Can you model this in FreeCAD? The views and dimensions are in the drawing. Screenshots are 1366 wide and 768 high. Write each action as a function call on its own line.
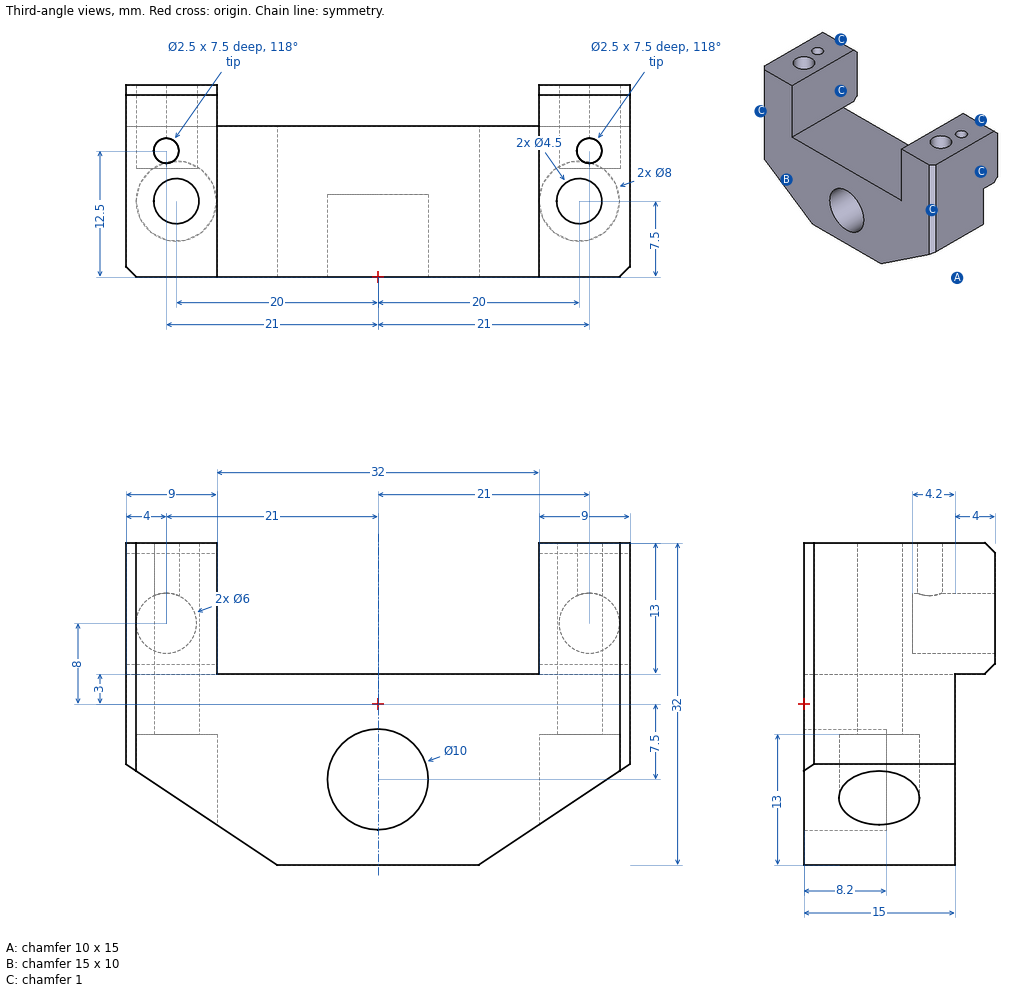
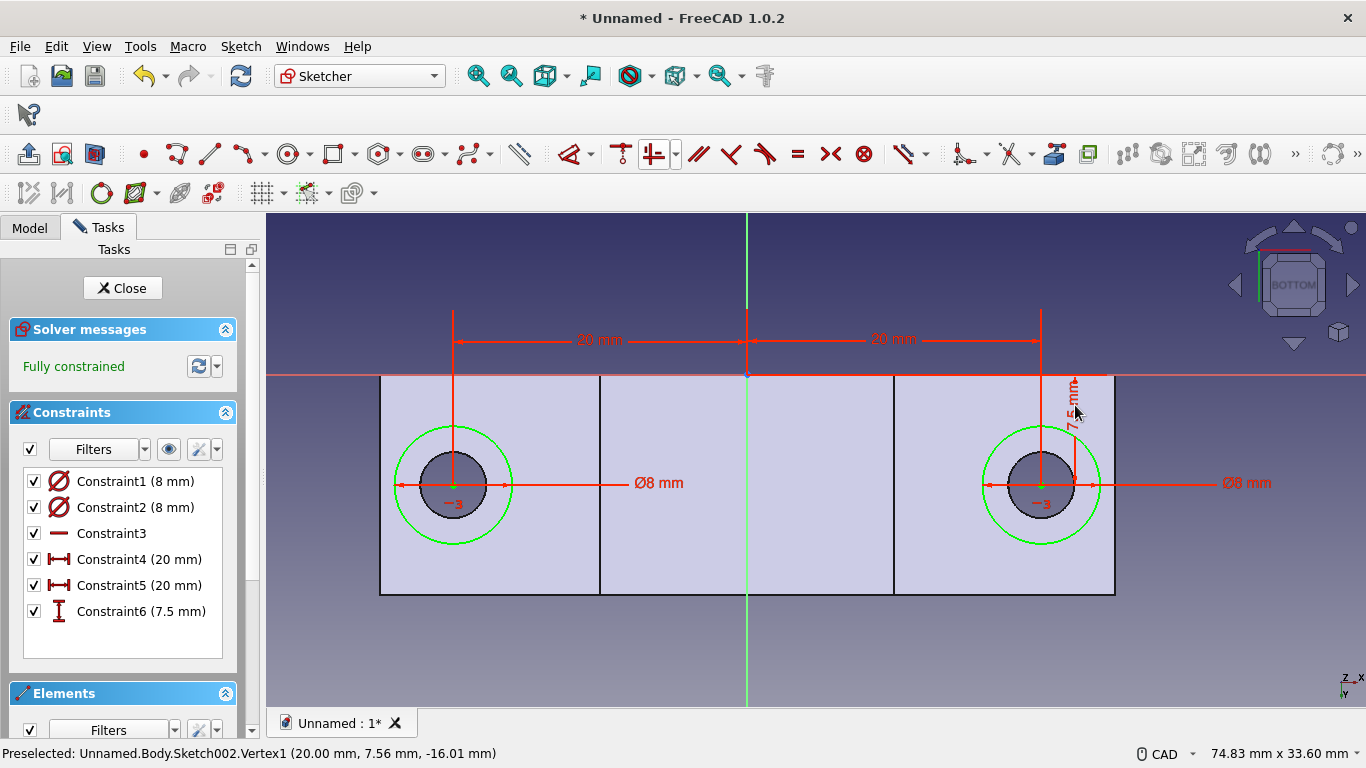
click(123, 288)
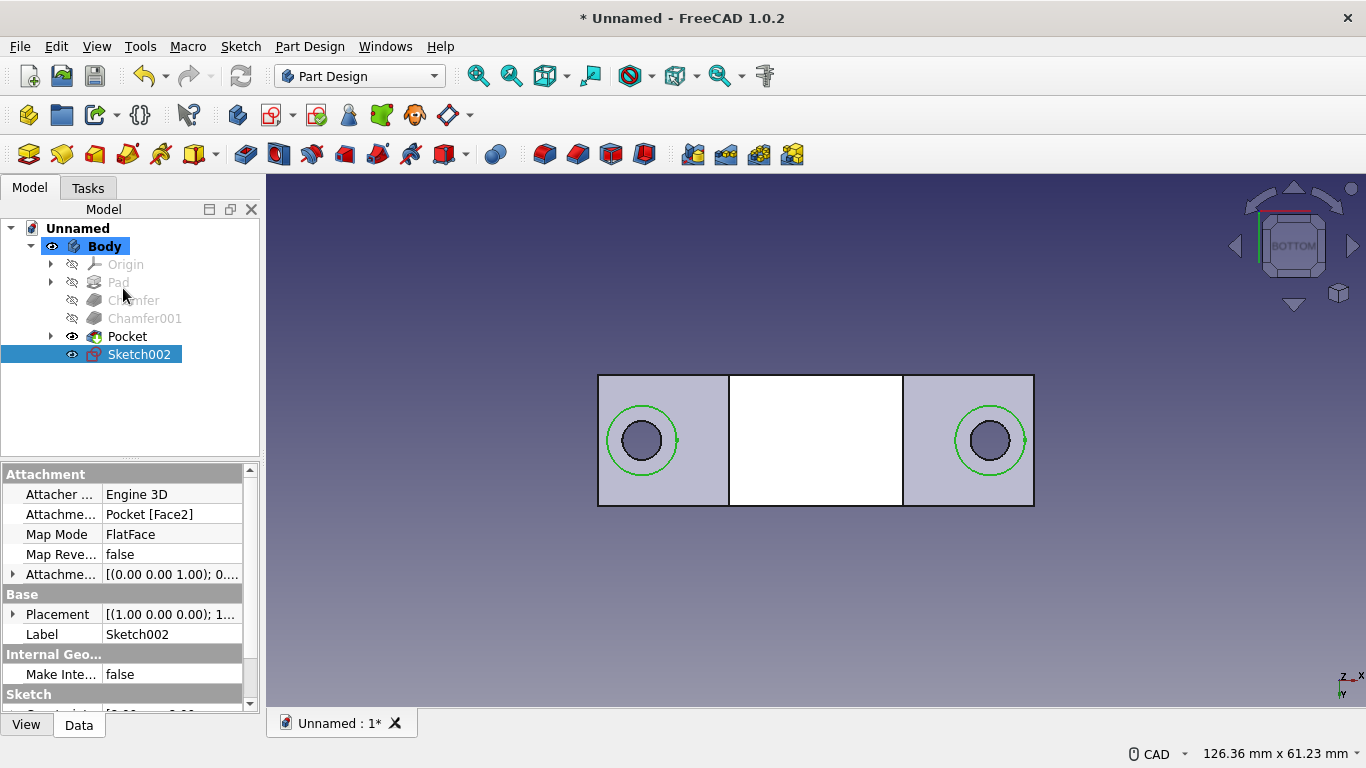
click(246, 154)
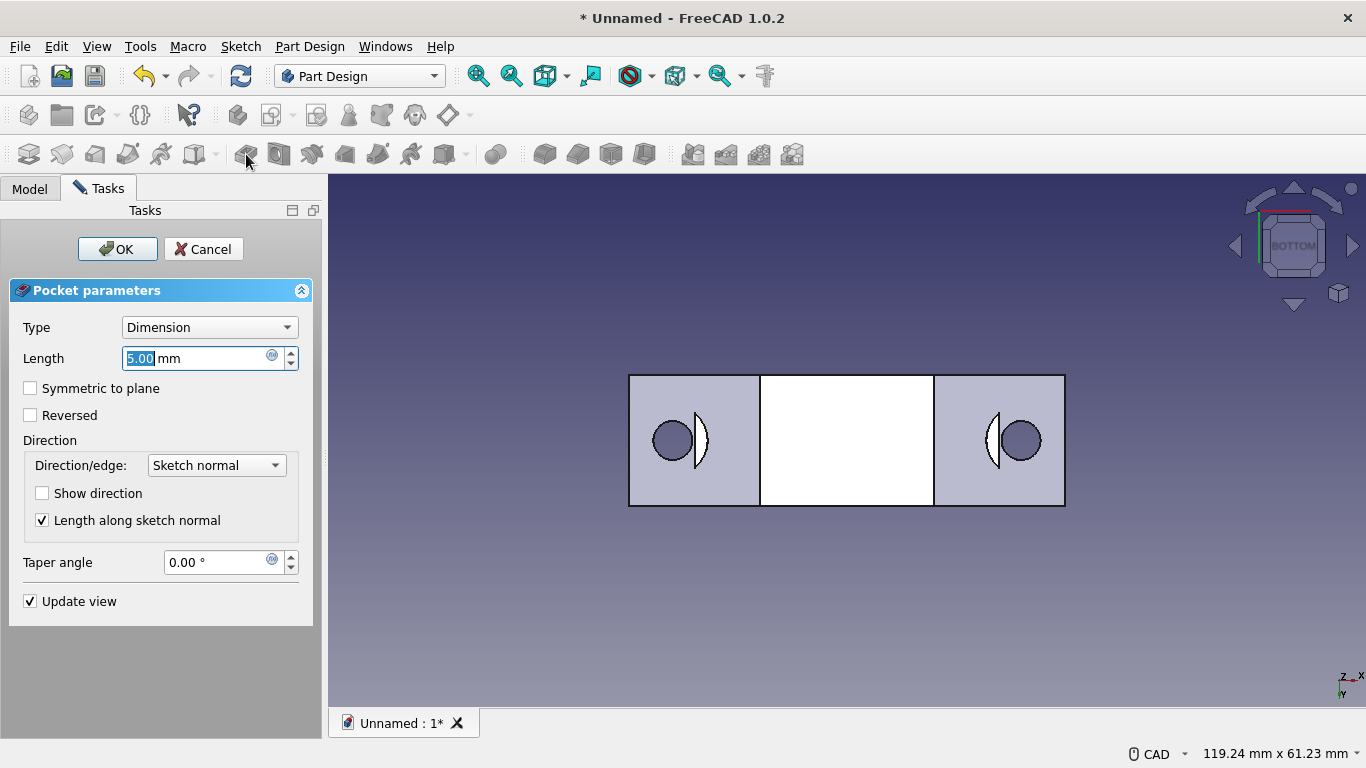
text(13)
key(Tab)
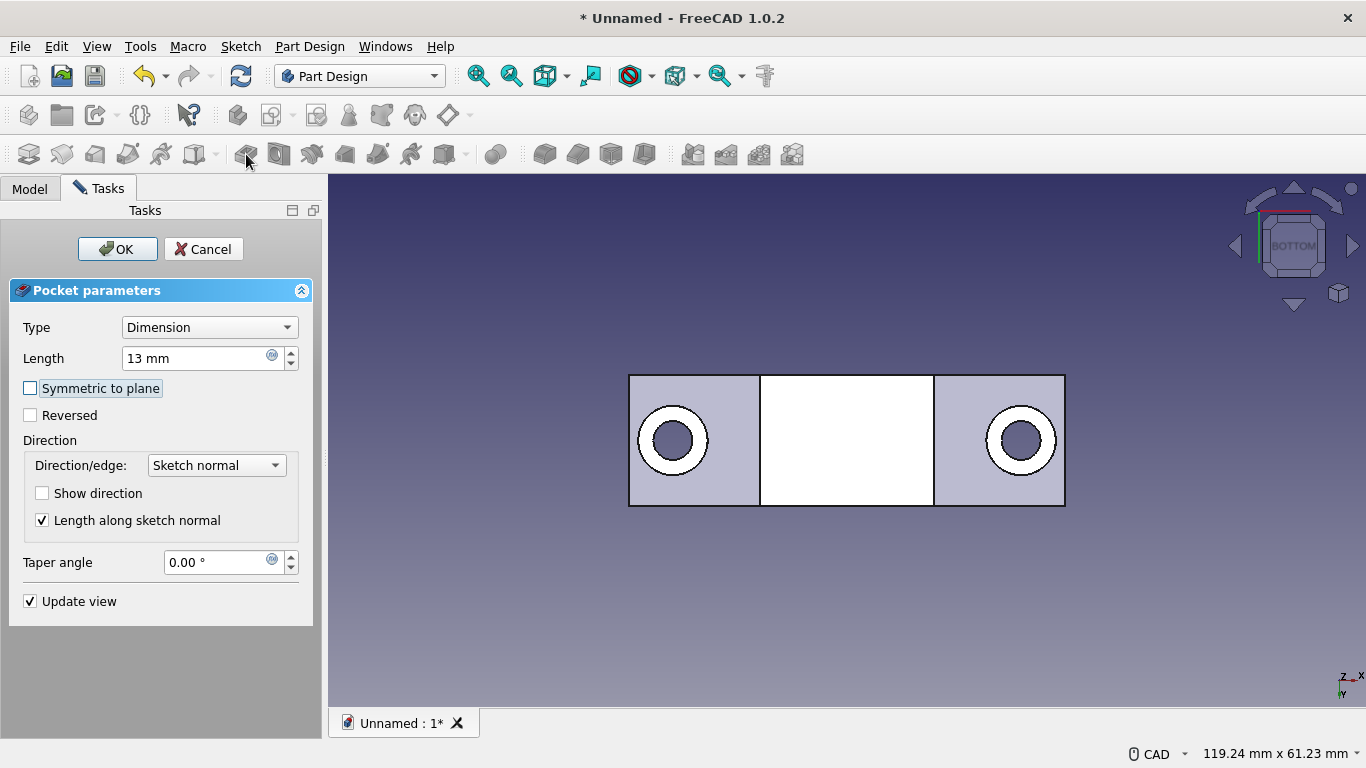
click(118, 249)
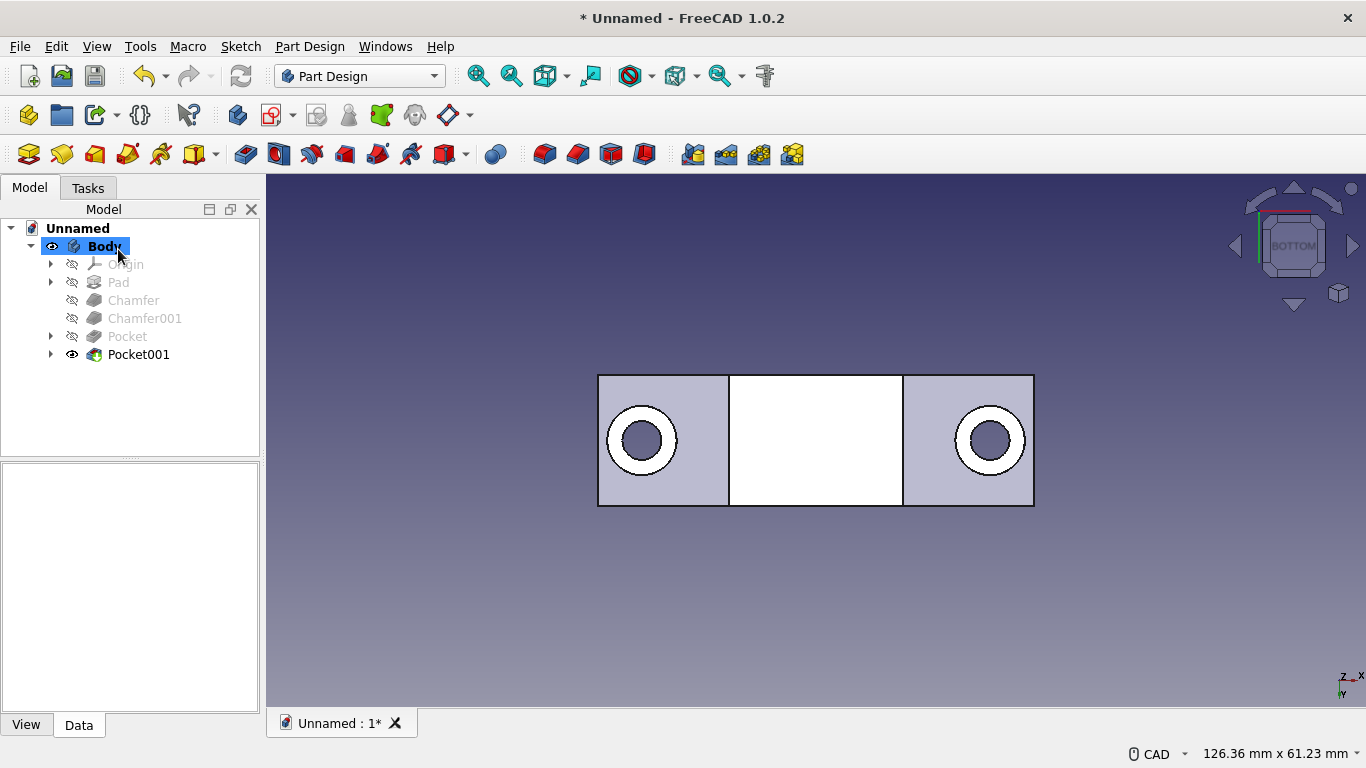
click(479, 76)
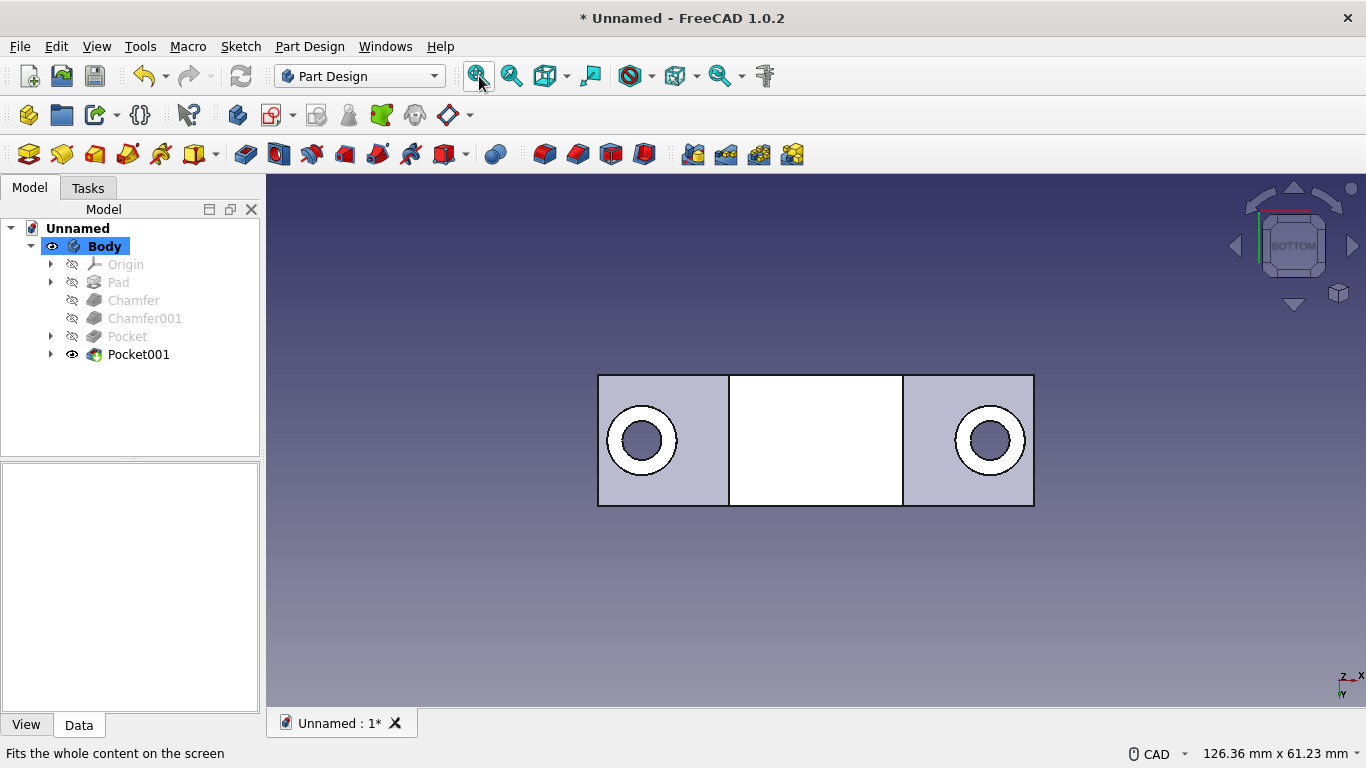
key(4)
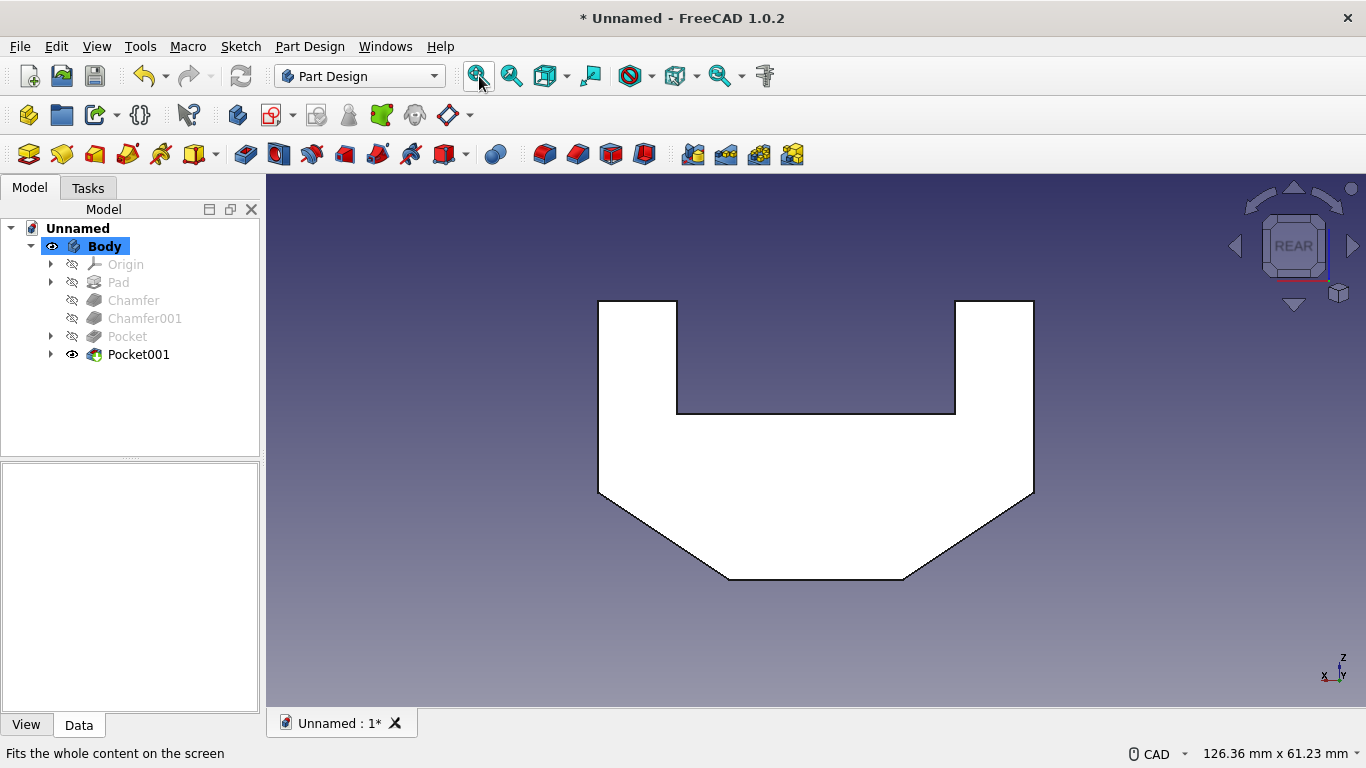
click(754, 479)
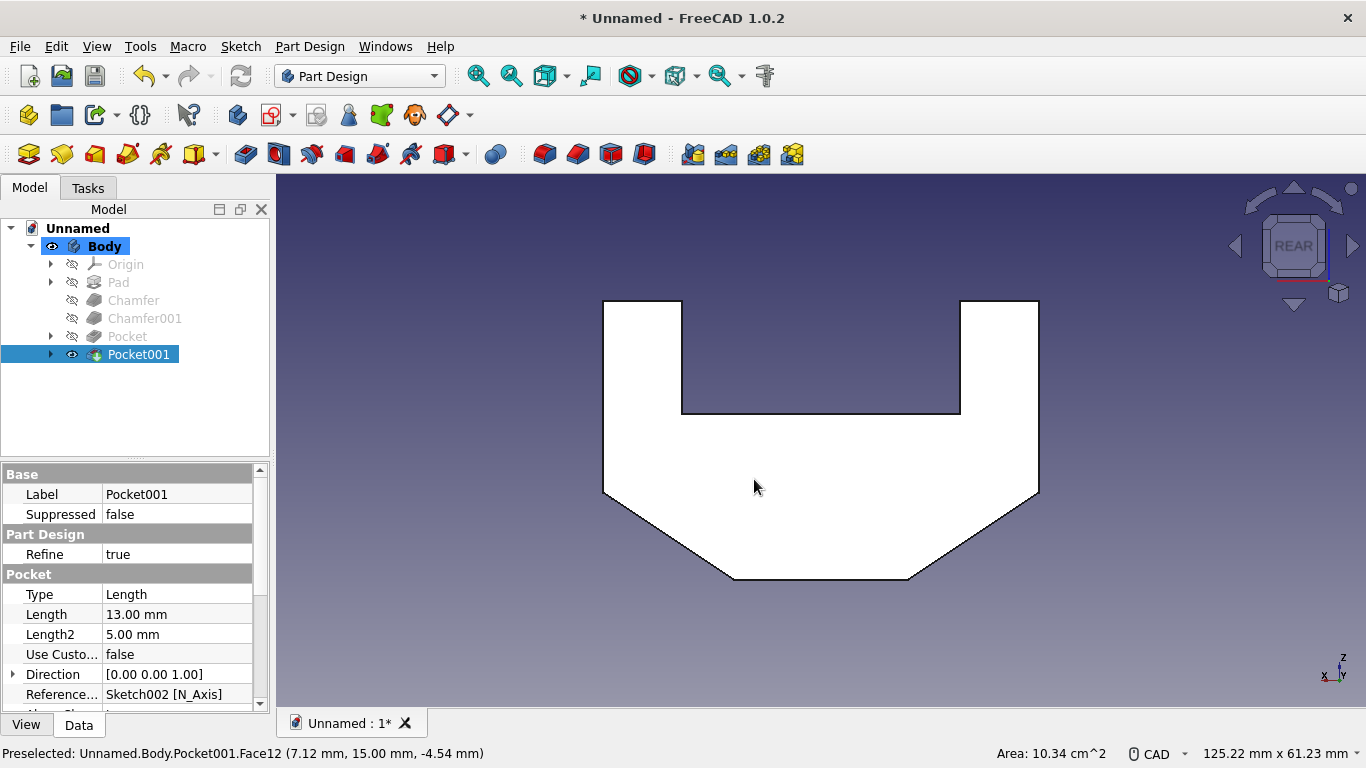
click(270, 116)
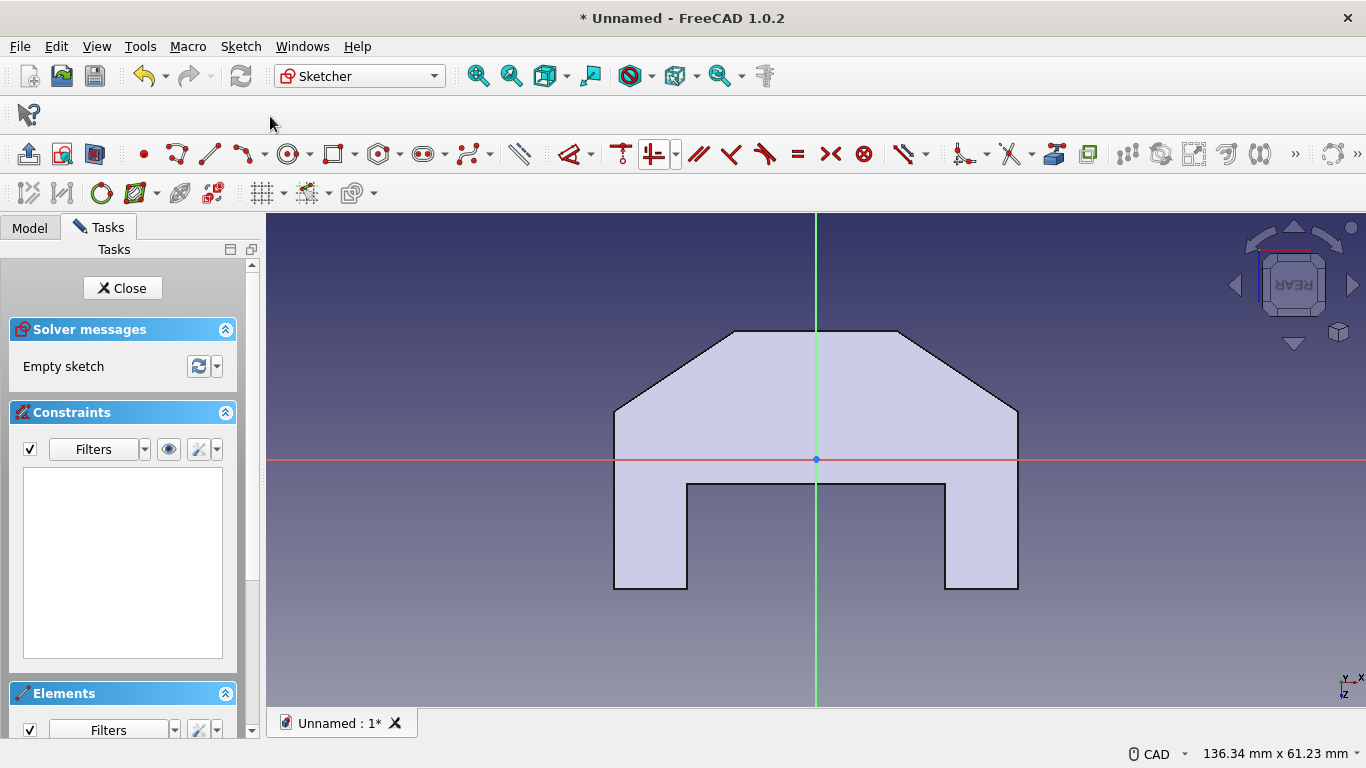
scroll(899, 558, up, 3)